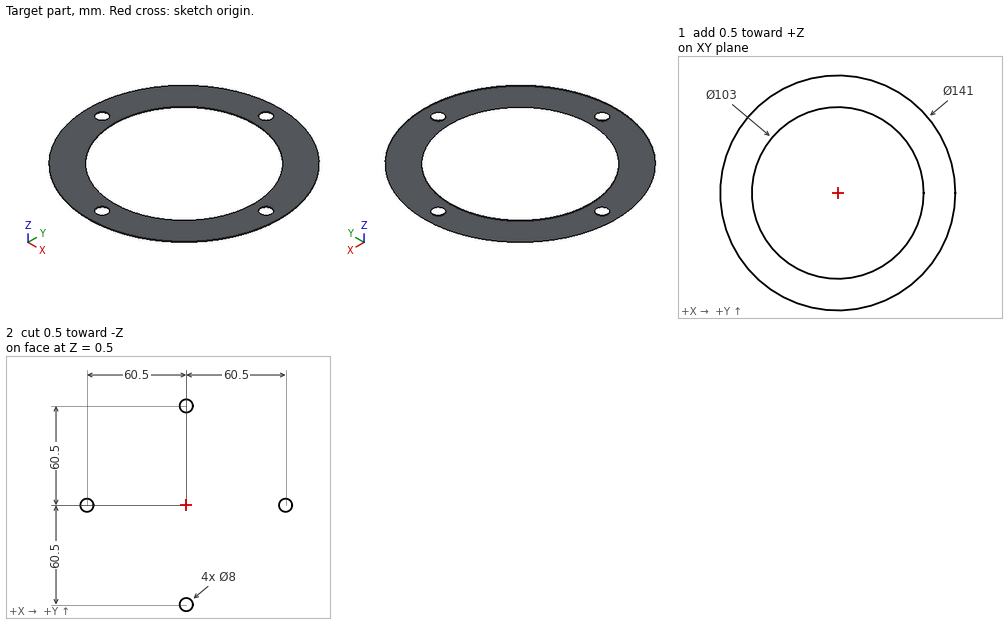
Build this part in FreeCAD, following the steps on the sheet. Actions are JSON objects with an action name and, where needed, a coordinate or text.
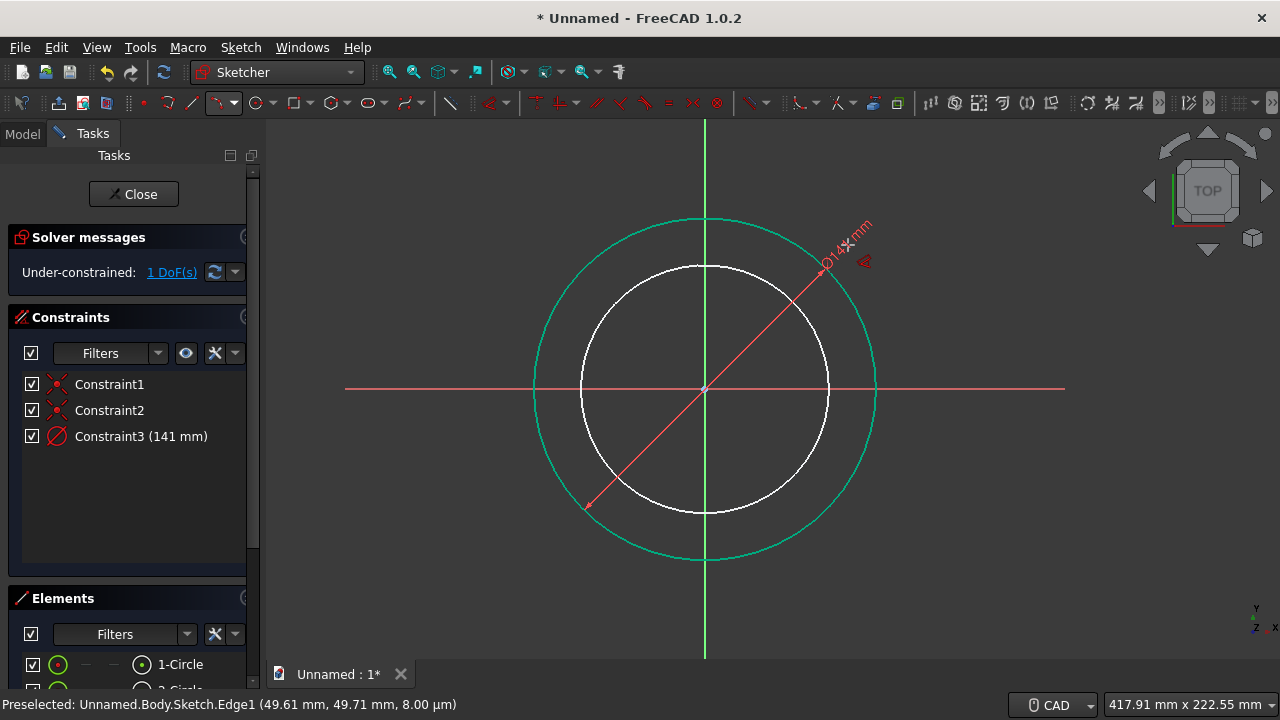
{"action": "left_click", "coordinate": [792, 301]}
{"action": "left_click", "coordinate": [814, 278]}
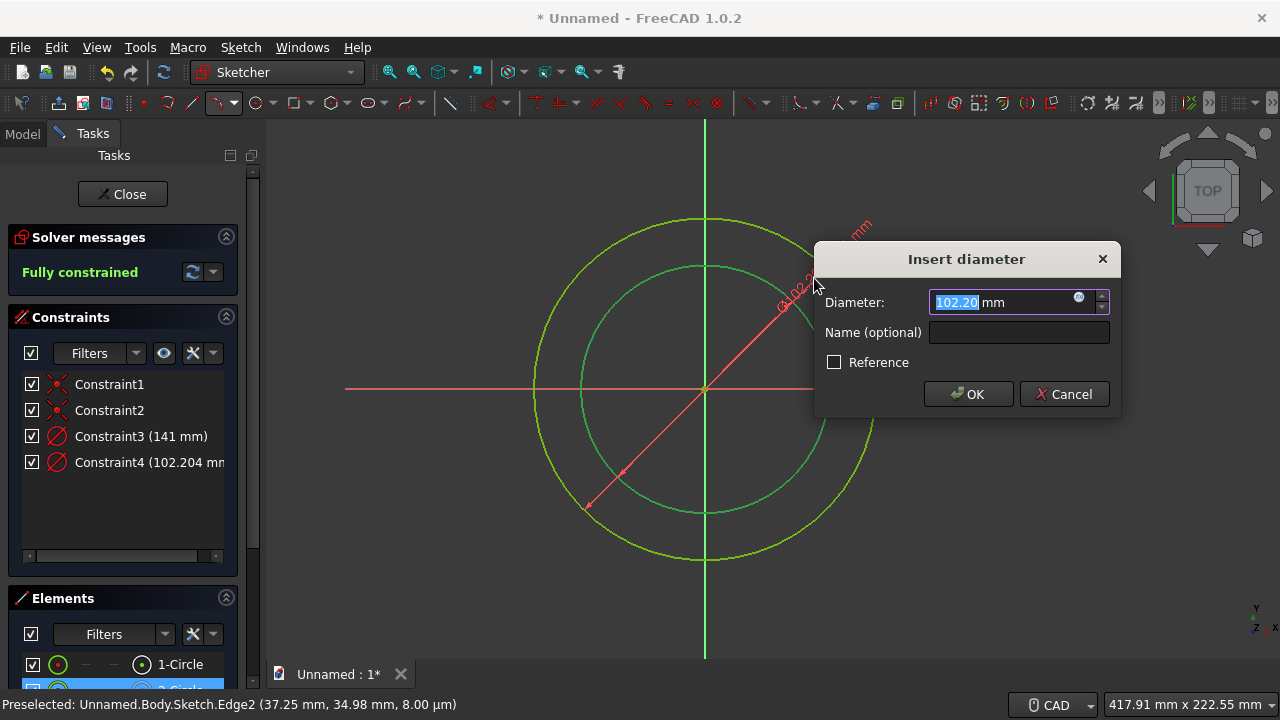
{"action": "type", "text": "103"}
{"action": "key", "text": "Return"}
{"action": "key", "text": "Escape"}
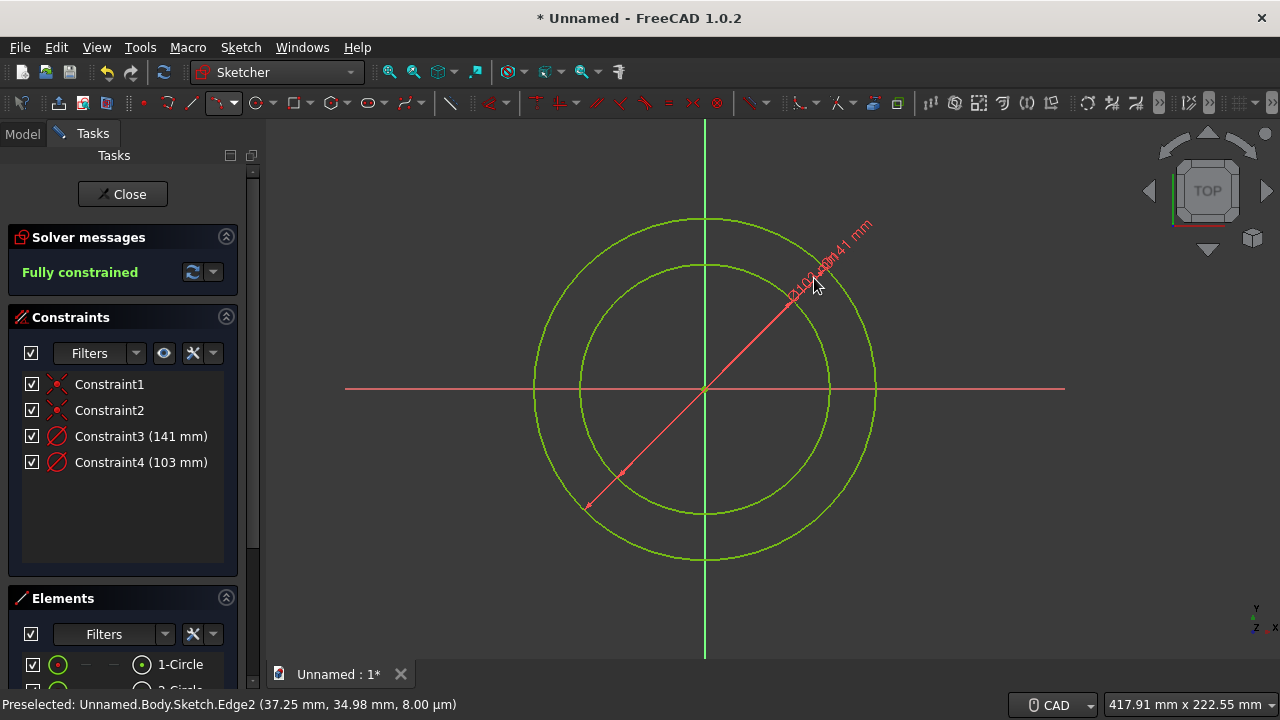
{"action": "left_click", "coordinate": [123, 194]}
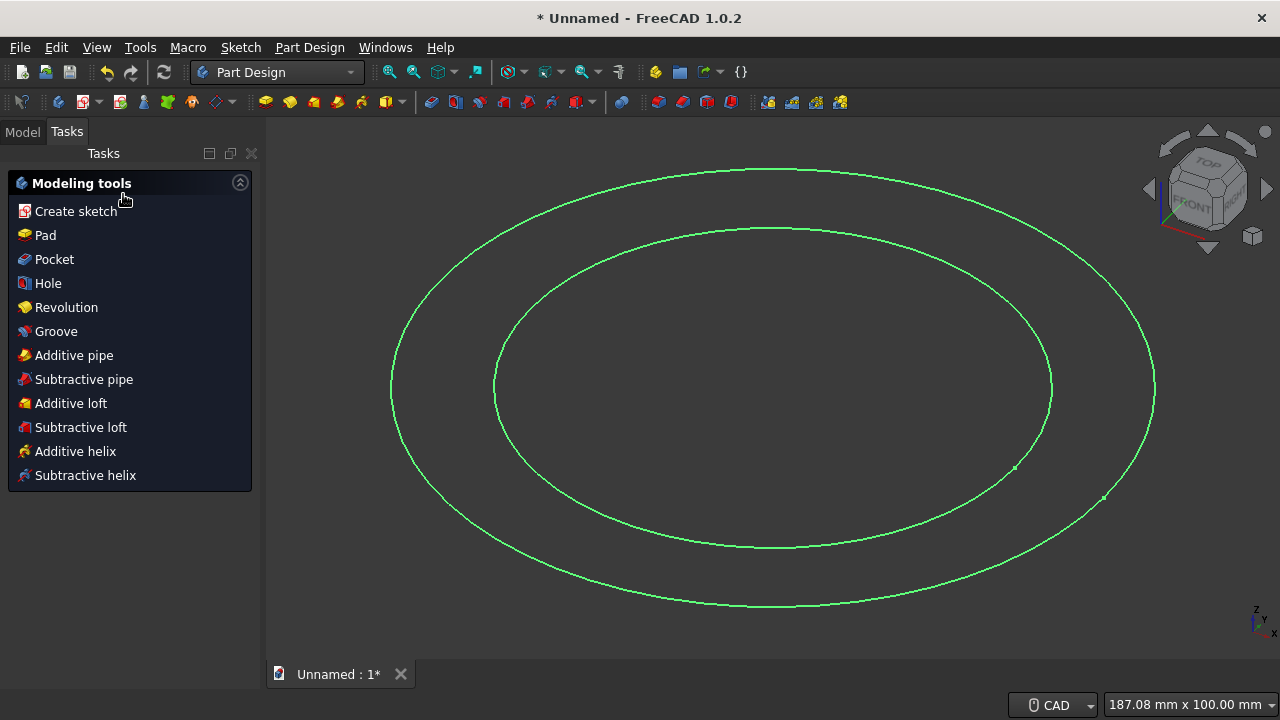
{"action": "left_click", "coordinate": [266, 102]}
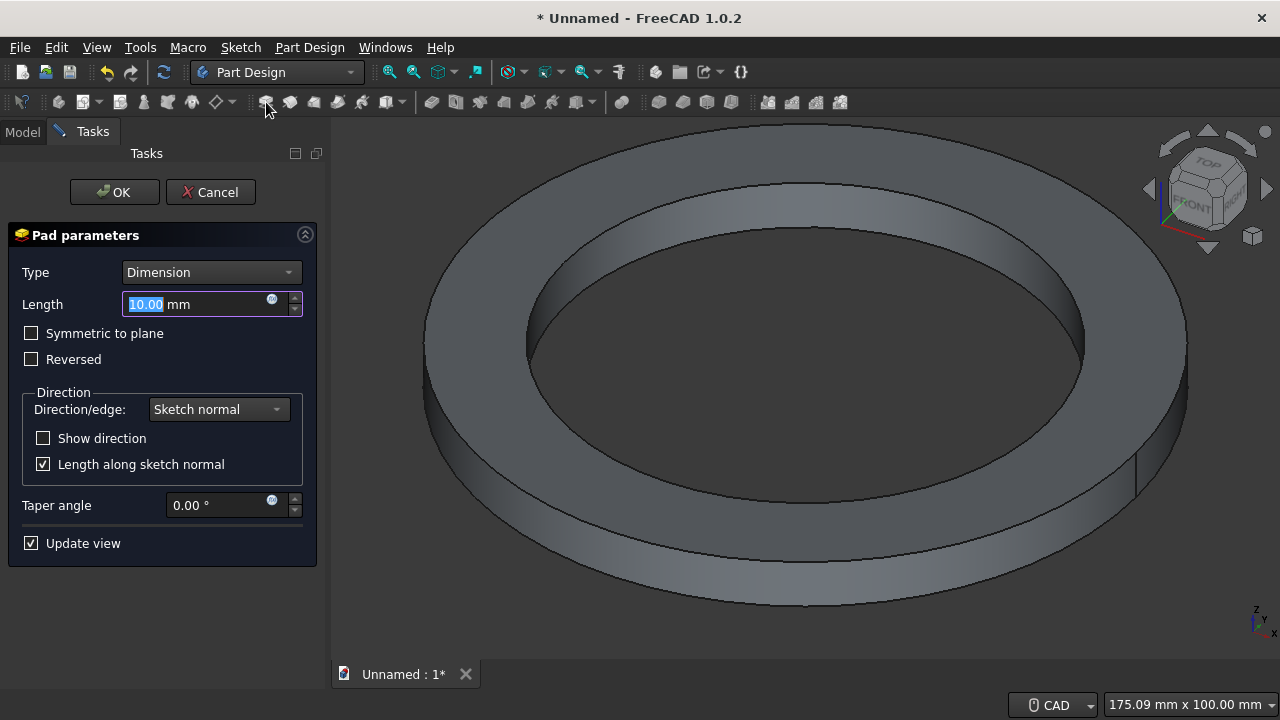
{"action": "type", "text": "0.5"}
{"action": "key", "text": "Tab"}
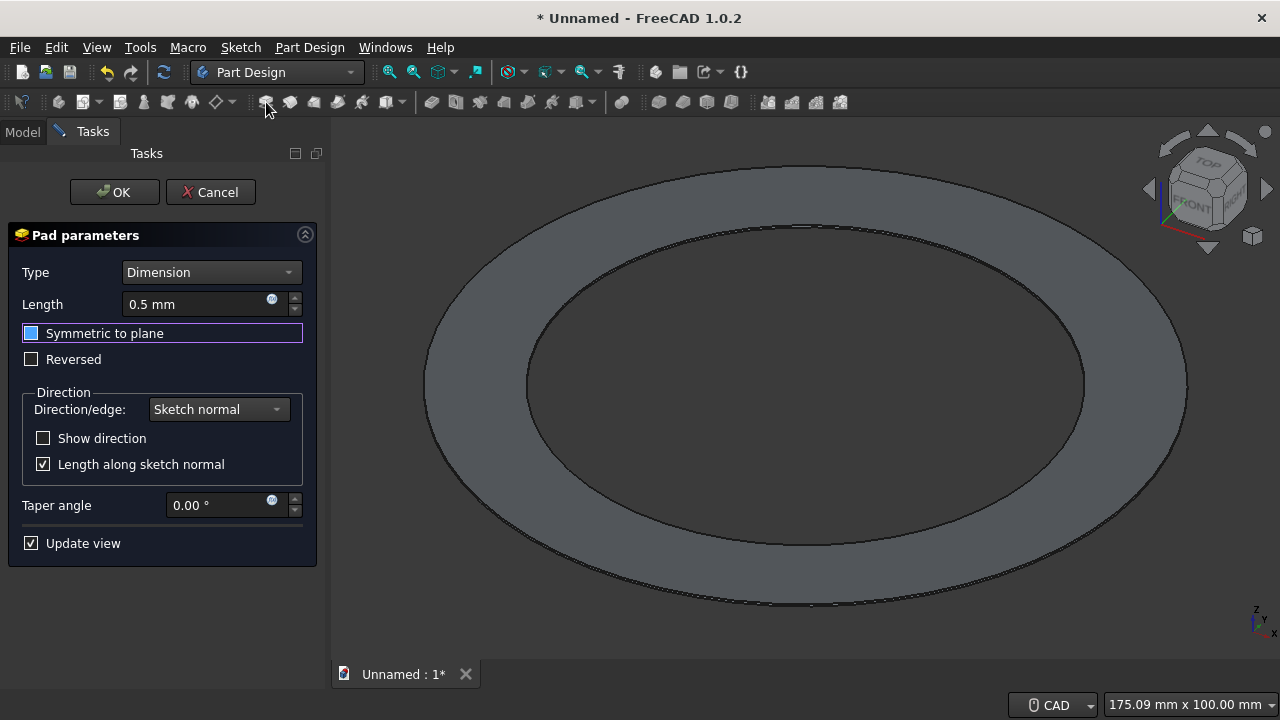
{"action": "left_click", "coordinate": [115, 192]}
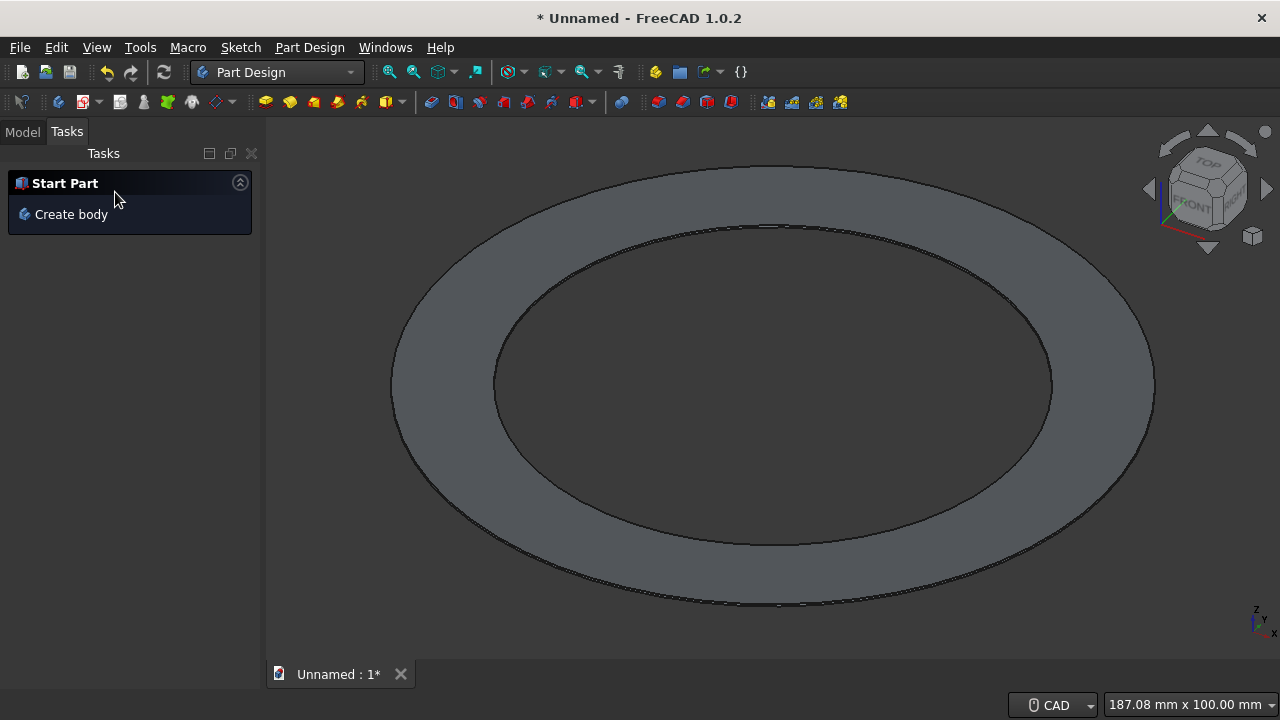
{"action": "left_click", "coordinate": [390, 72]}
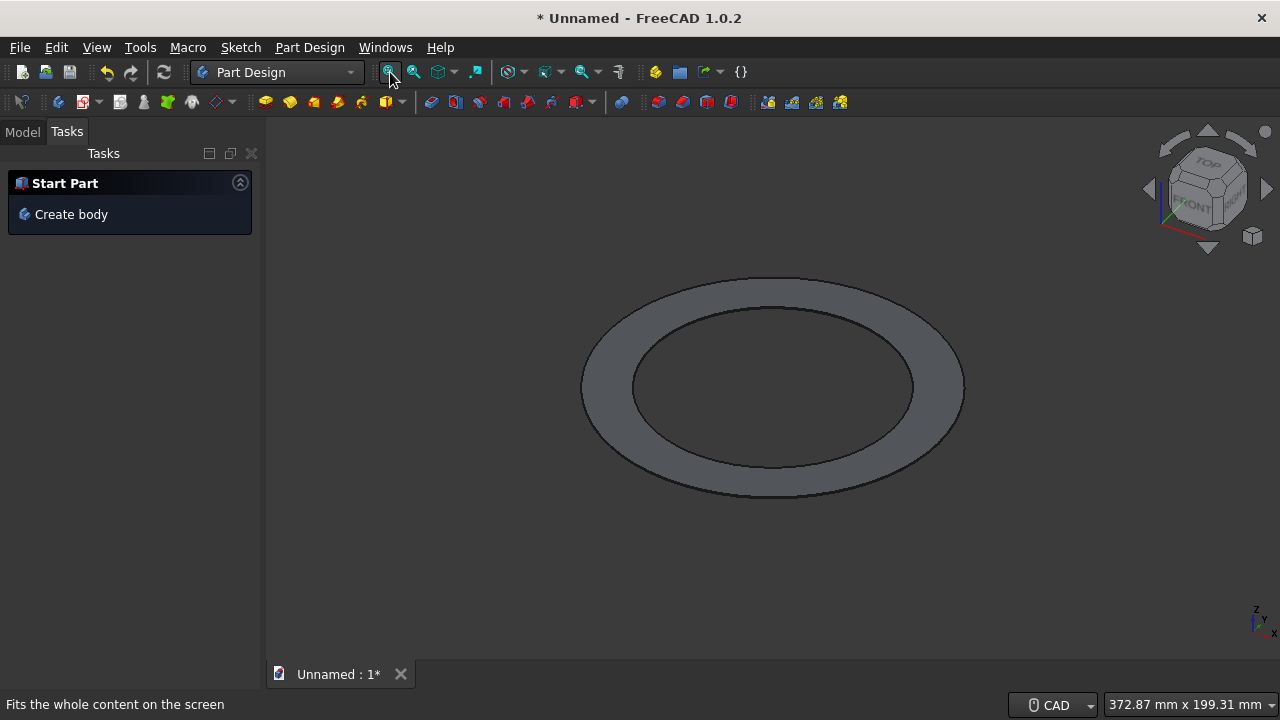
{"action": "left_click", "coordinate": [691, 468]}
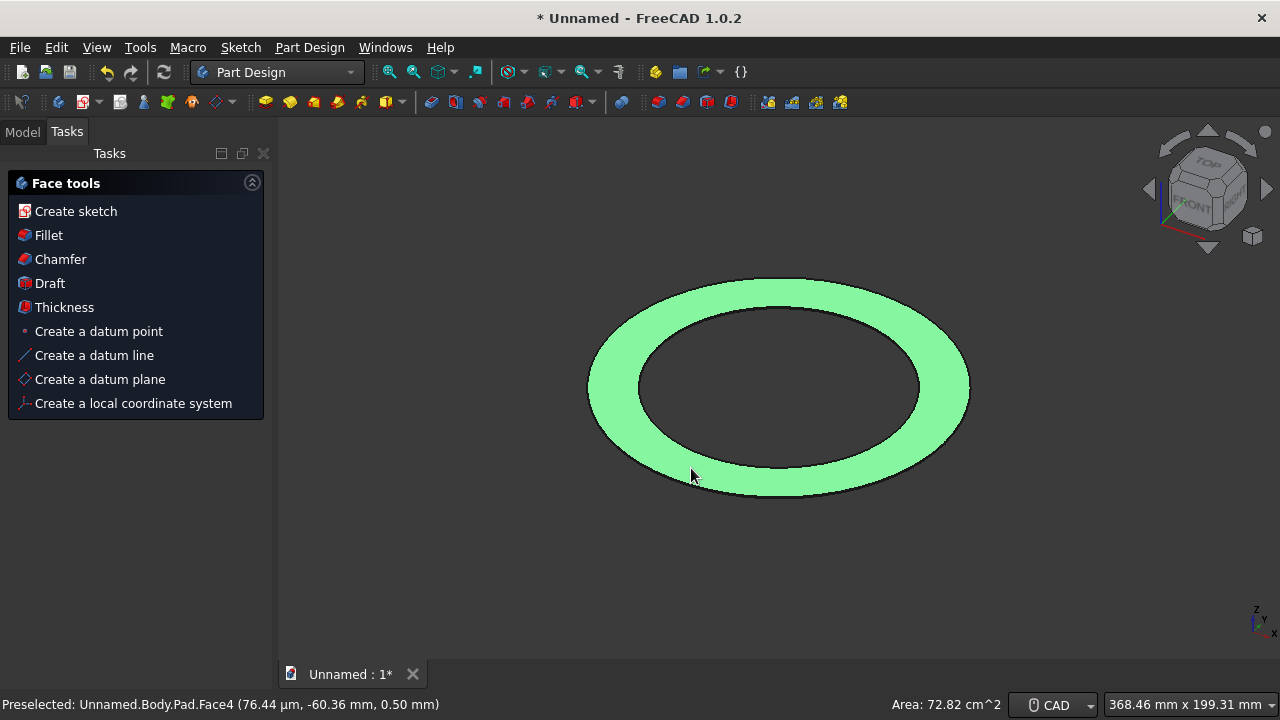
{"action": "left_click", "coordinate": [84, 102]}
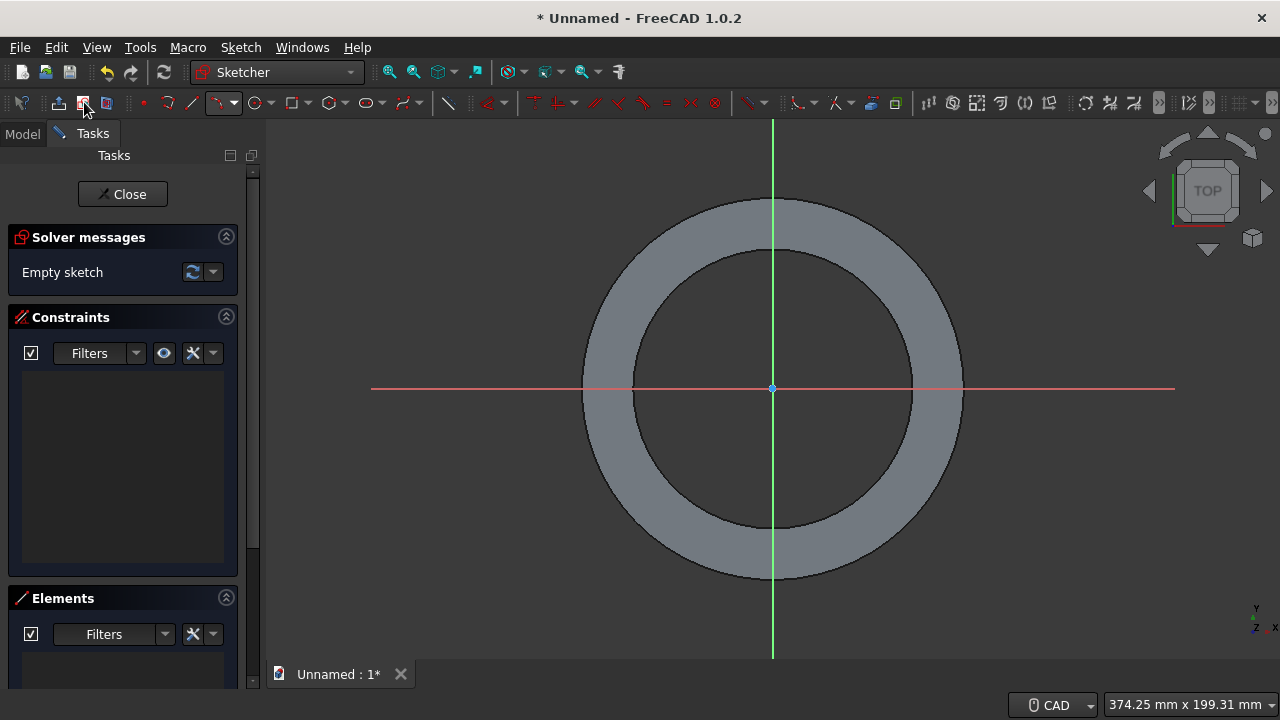
{"action": "left_click", "coordinate": [256, 104]}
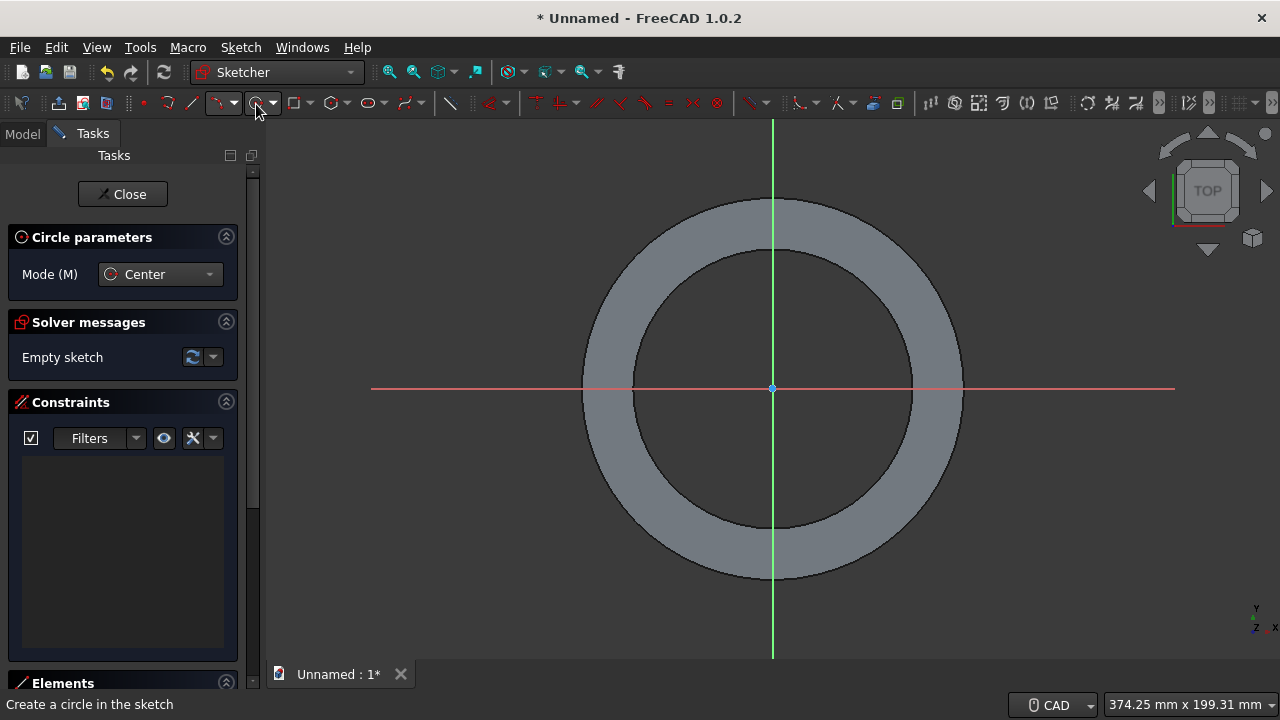
{"action": "scroll", "coordinate": [773, 553], "scroll_direction": "up", "scroll_amount": 4}